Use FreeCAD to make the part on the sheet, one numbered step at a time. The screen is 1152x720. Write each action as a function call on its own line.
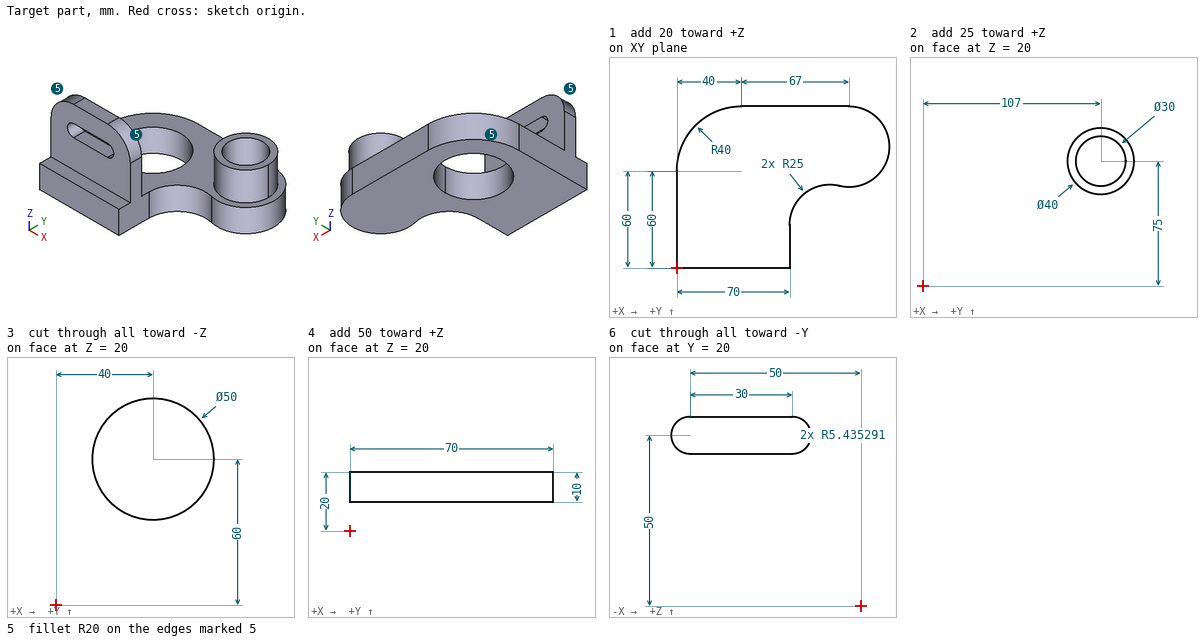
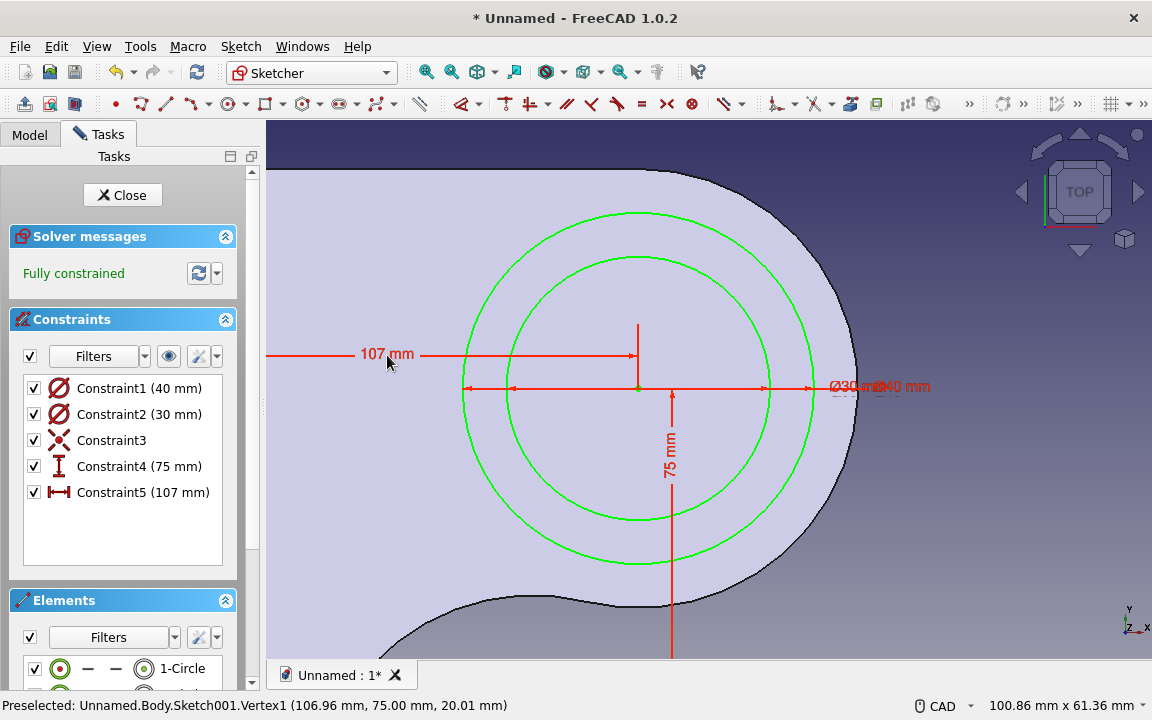
click(123, 195)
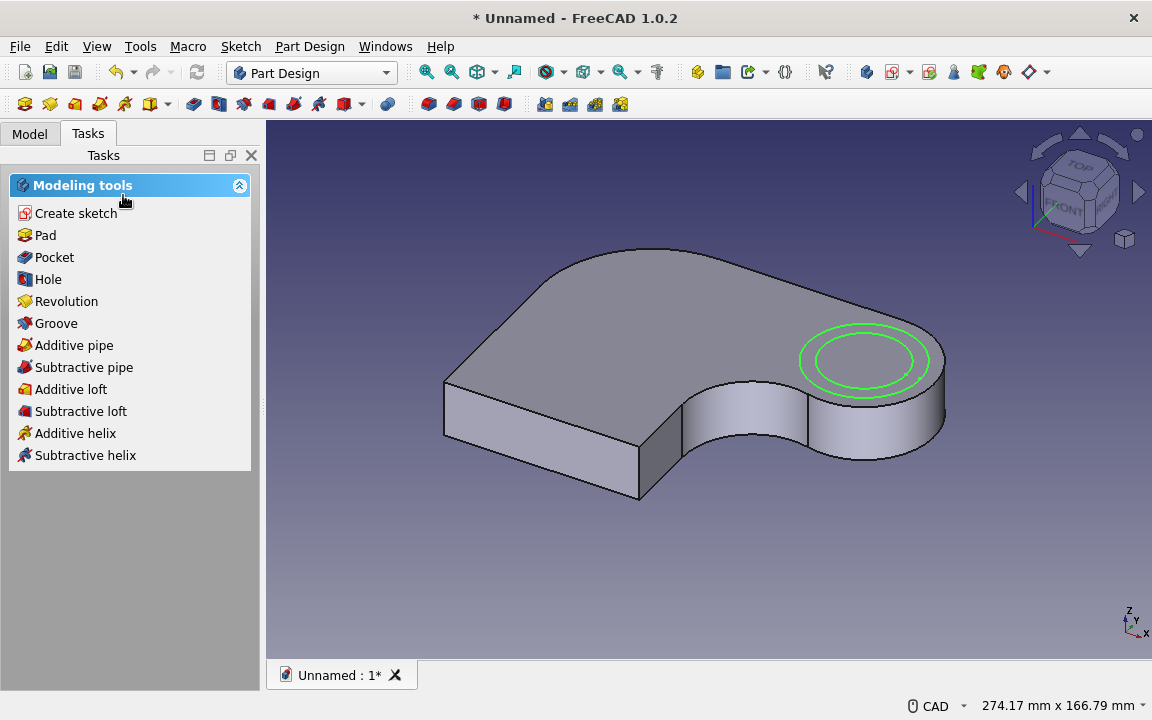
click(25, 104)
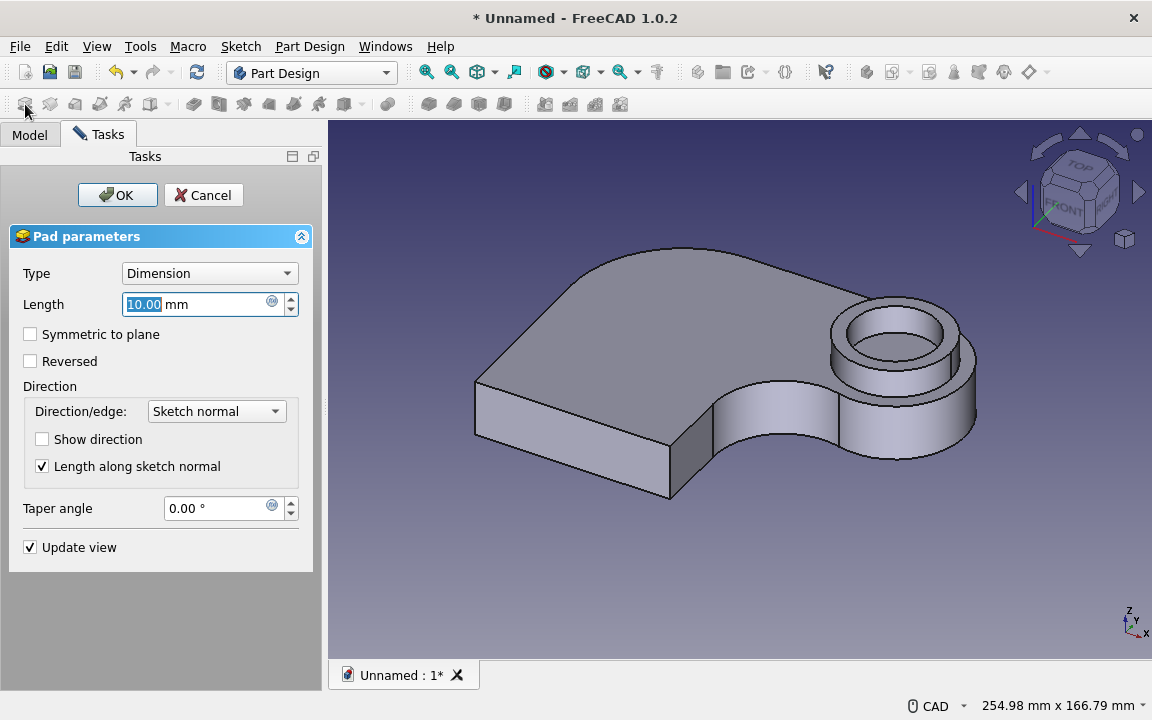
text(25)
key(Tab)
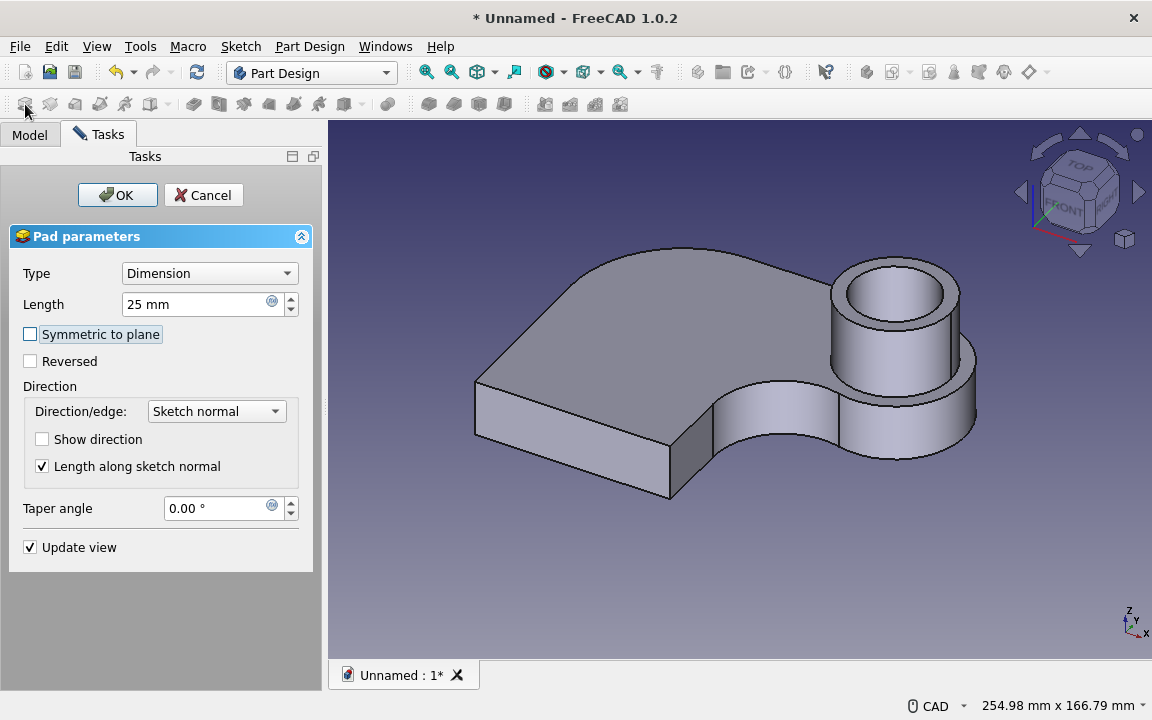
click(118, 195)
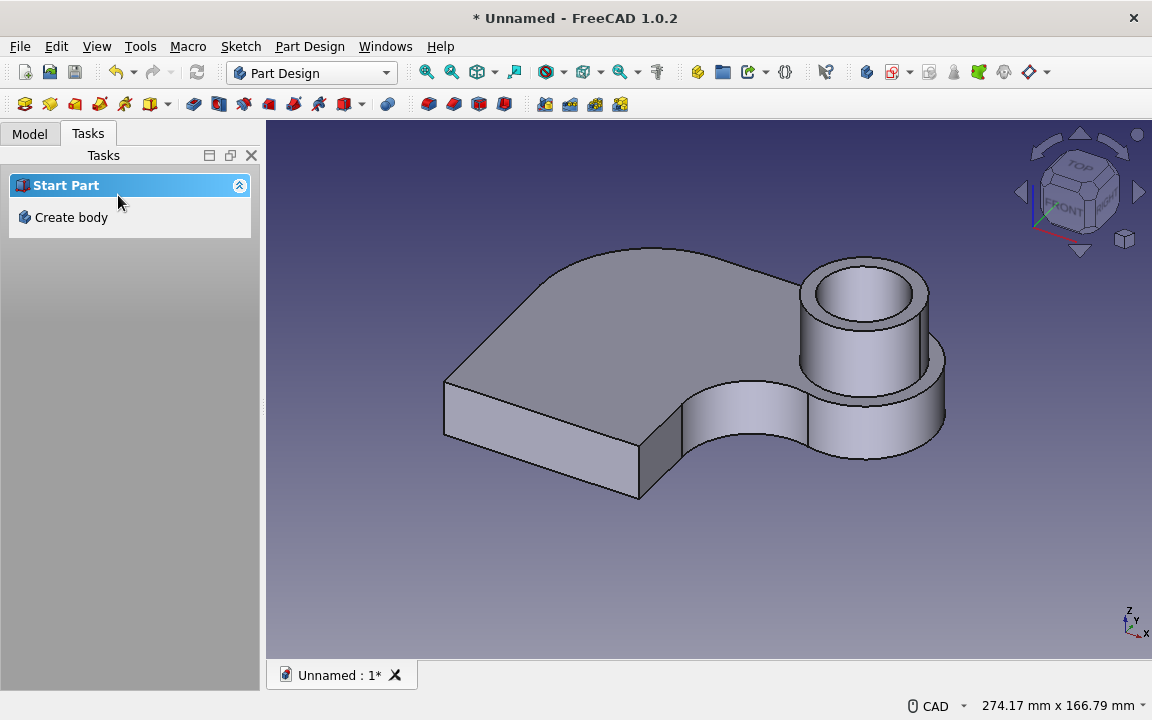
click(679, 321)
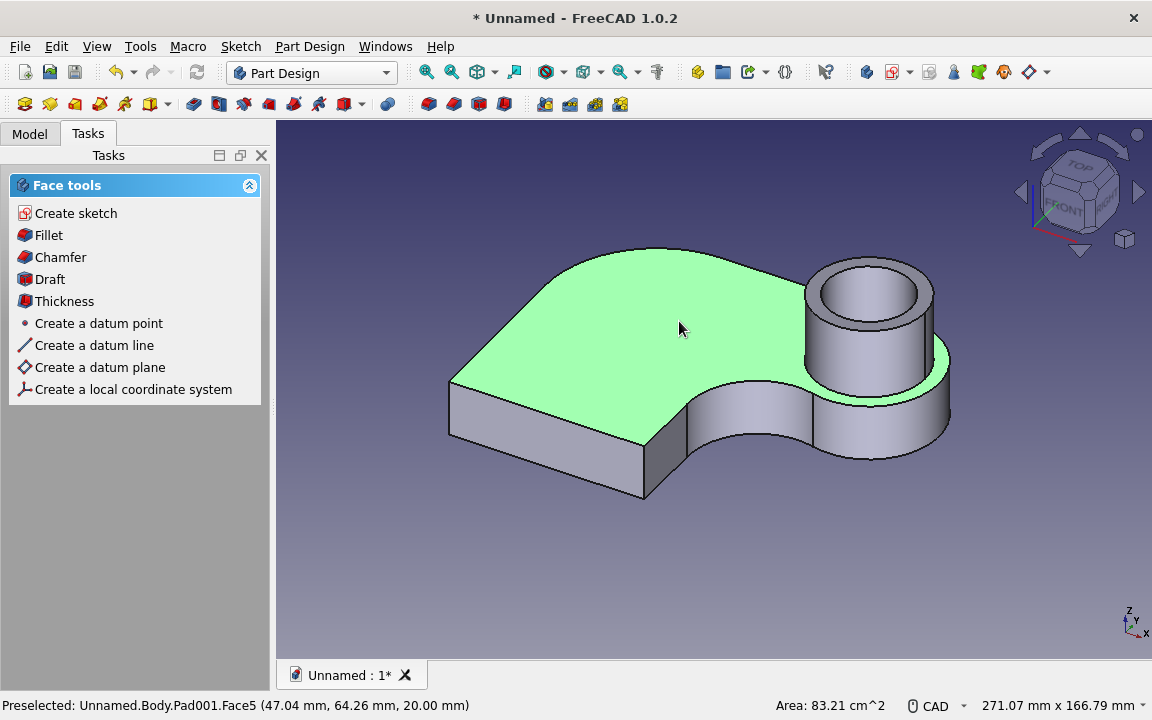
click(892, 72)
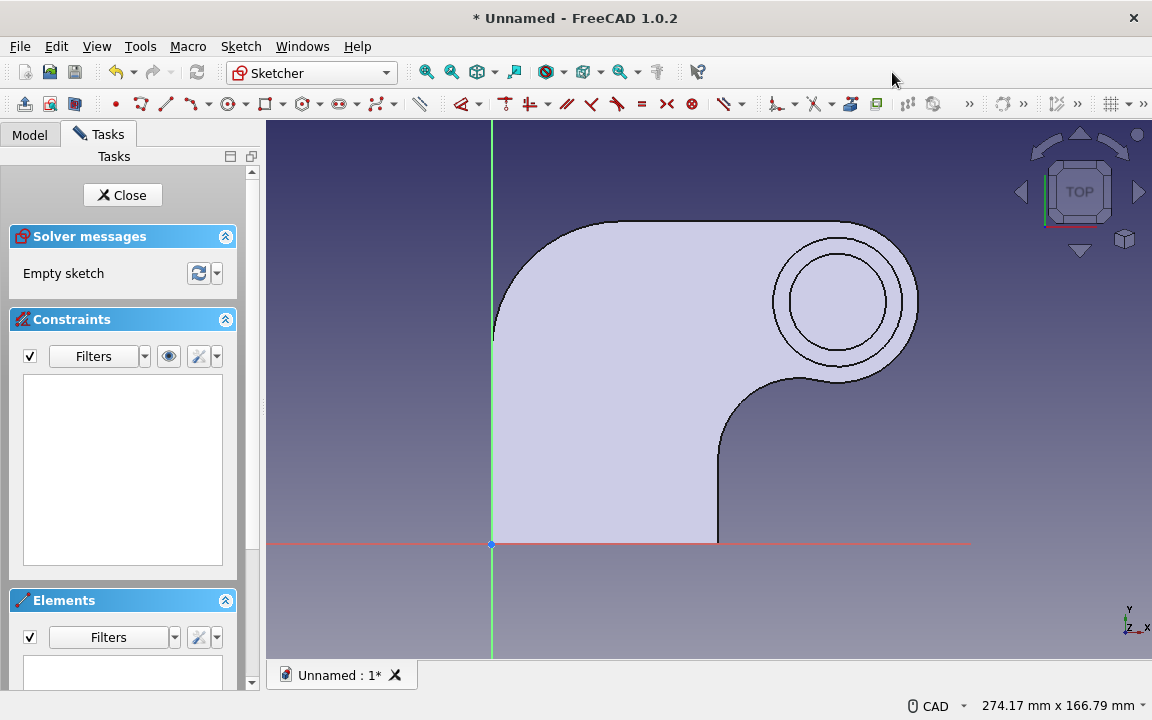
click(75, 104)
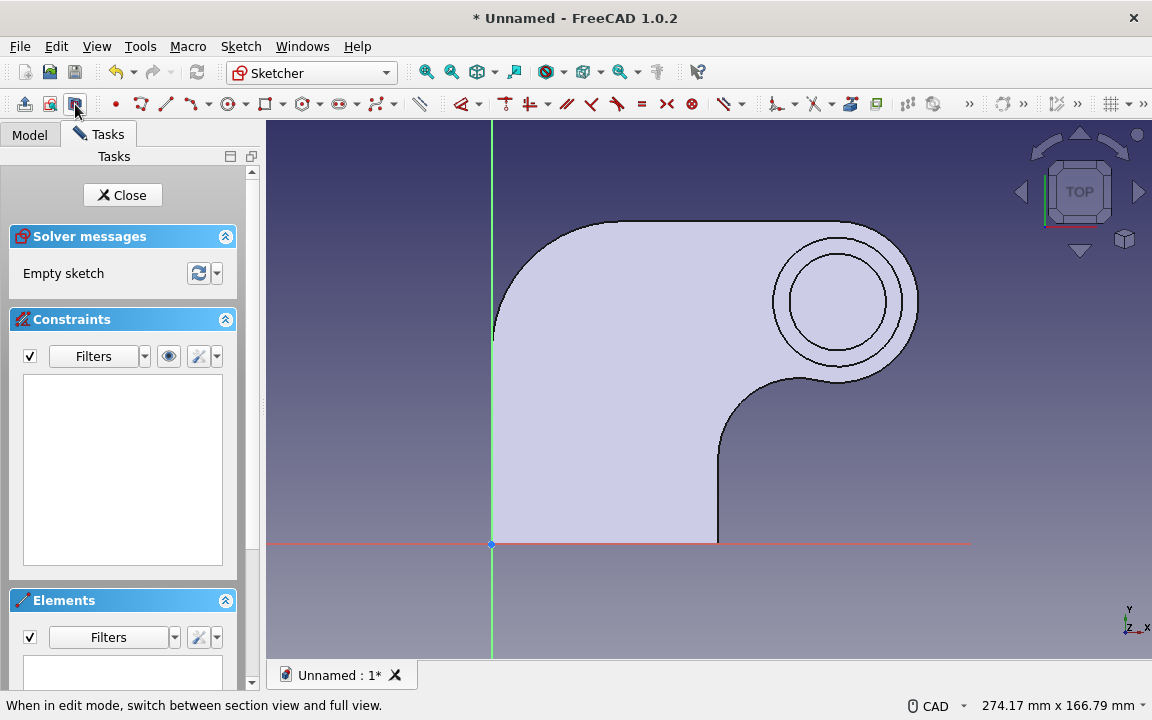
click(228, 104)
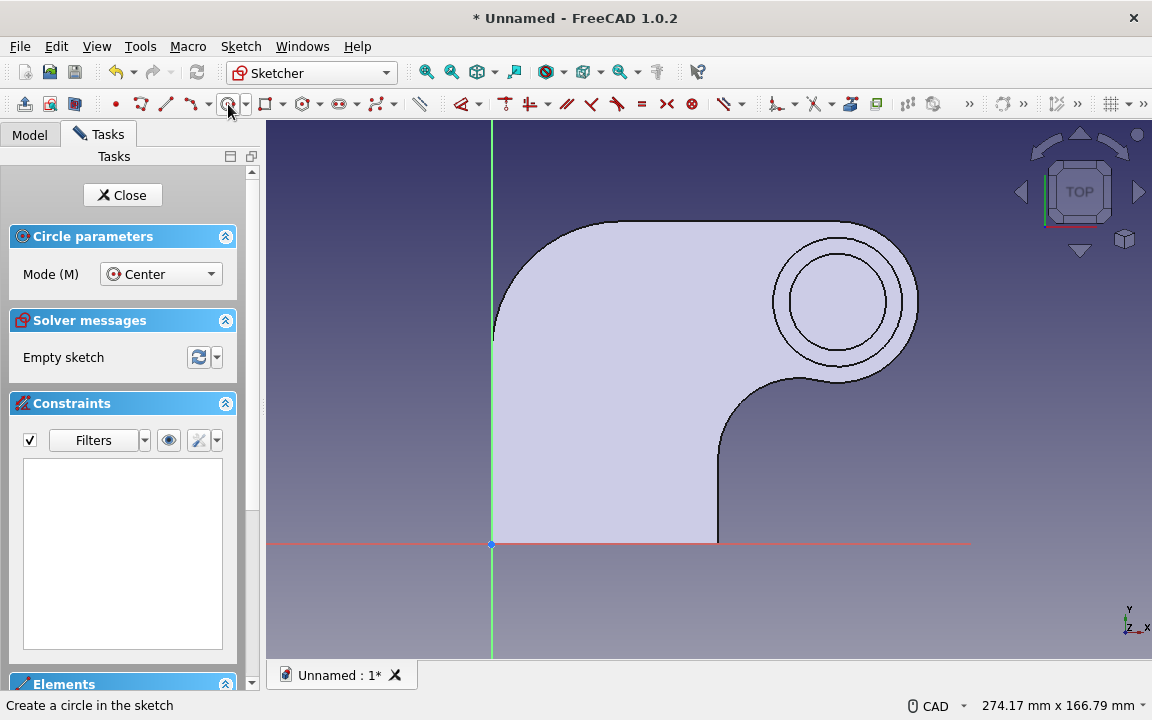
click(621, 351)
move(678, 293)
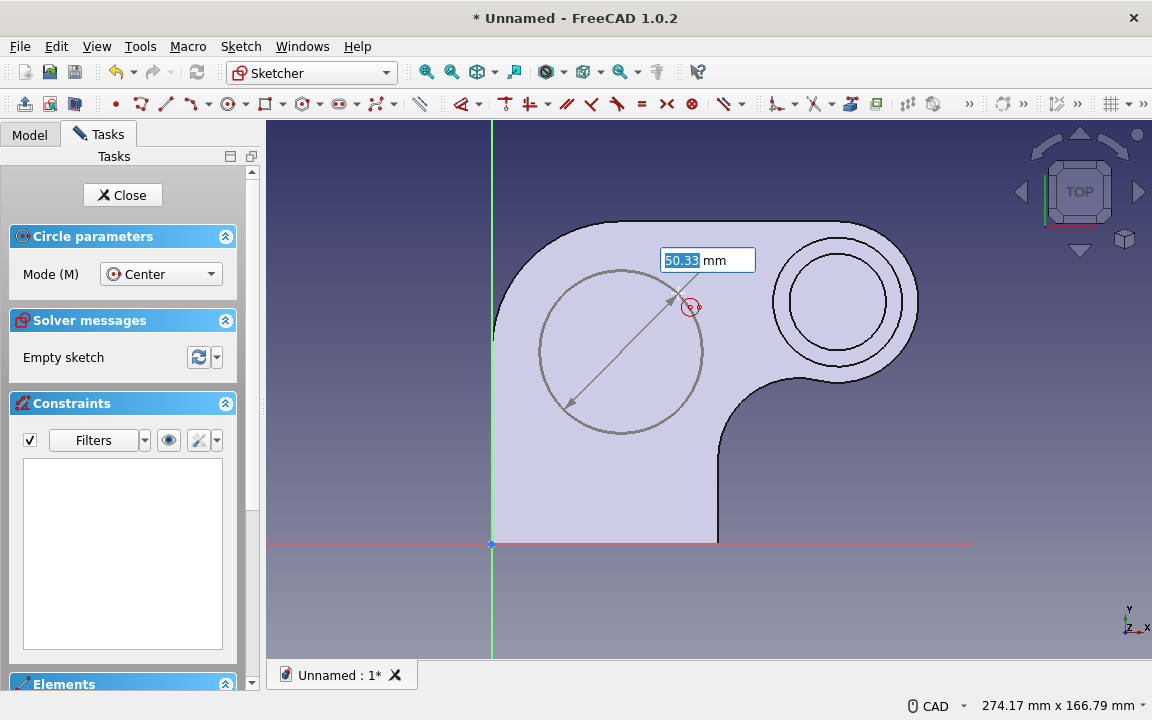
text(50)
key(Return)
key(Escape)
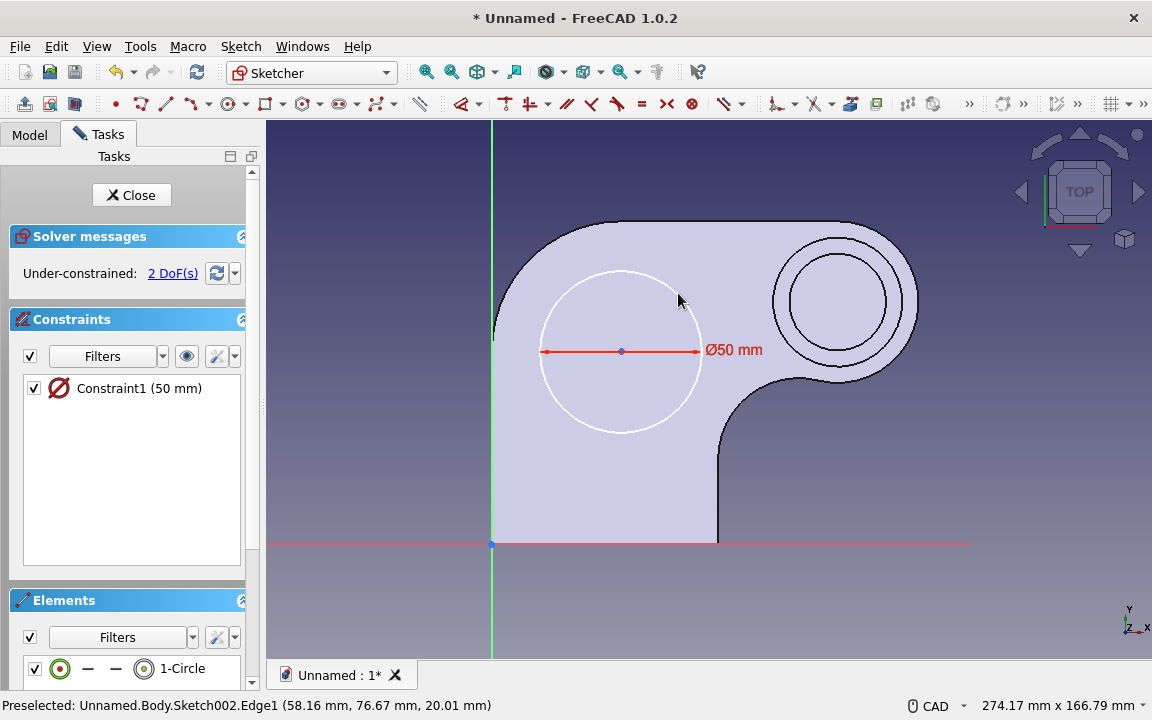
click(460, 104)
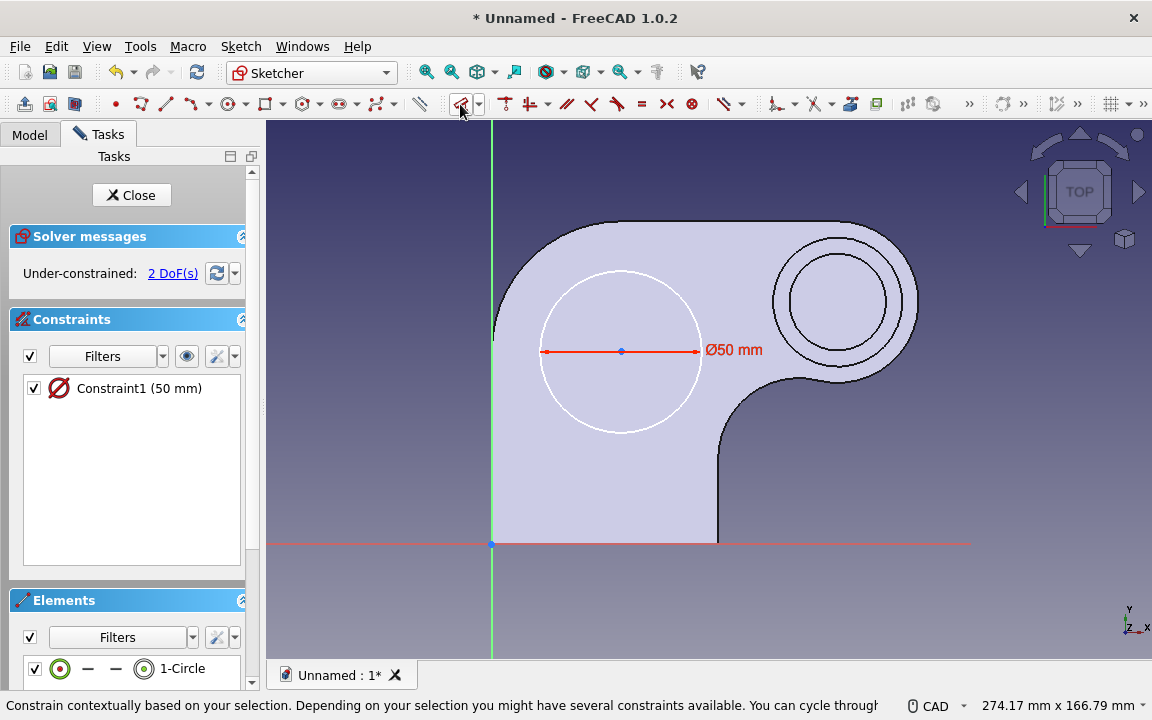
click(621, 352)
click(556, 578)